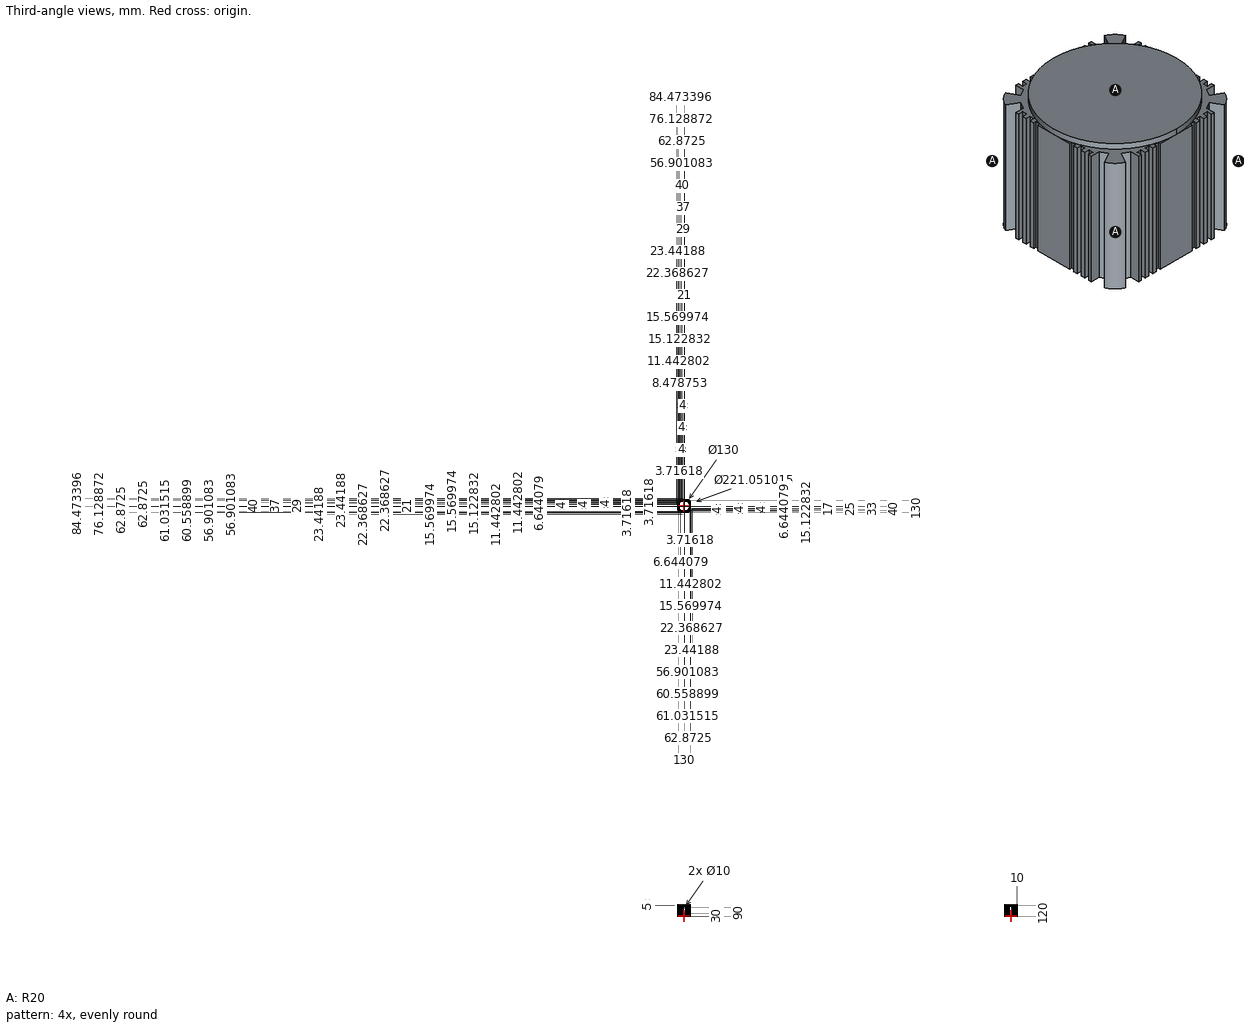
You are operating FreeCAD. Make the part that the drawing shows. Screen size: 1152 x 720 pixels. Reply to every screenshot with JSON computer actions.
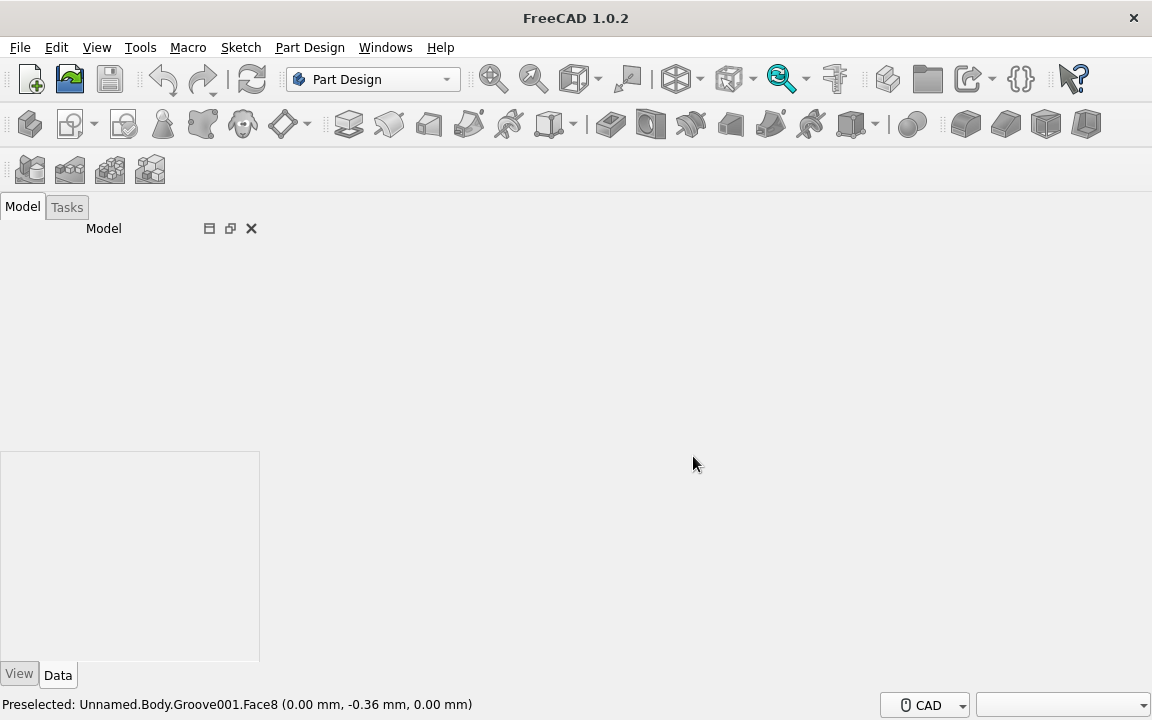
{"action": "key", "text": "ctrl+n"}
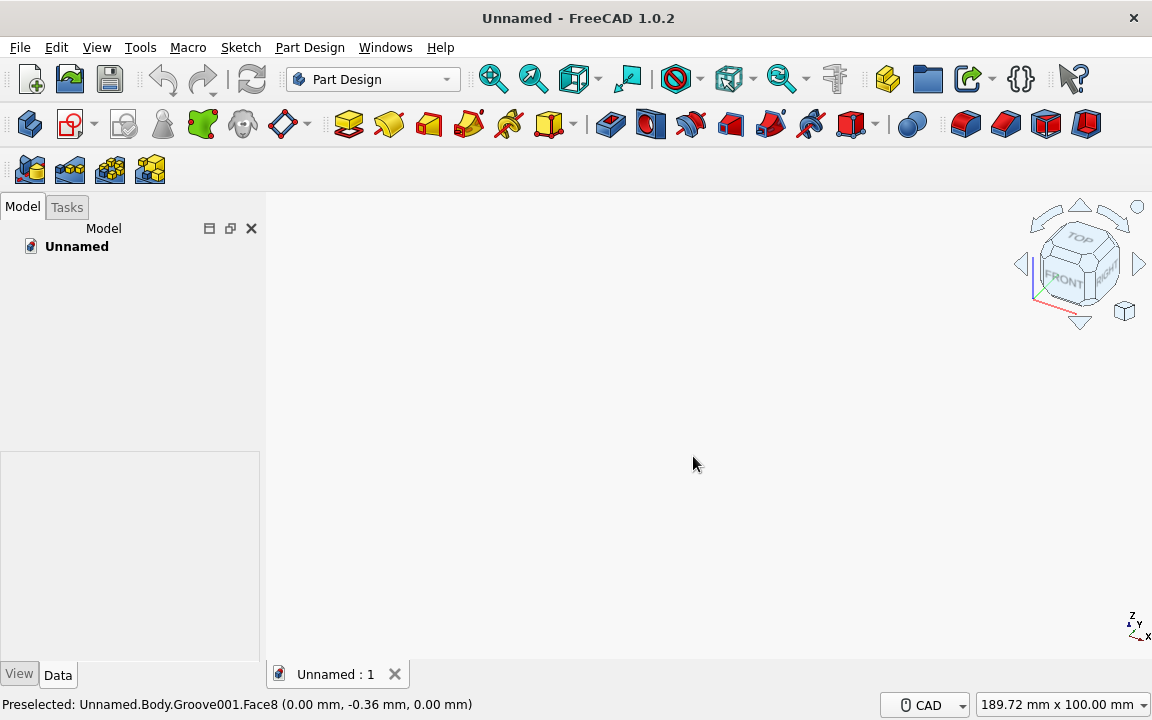
{"action": "left_click", "coordinate": [70, 124]}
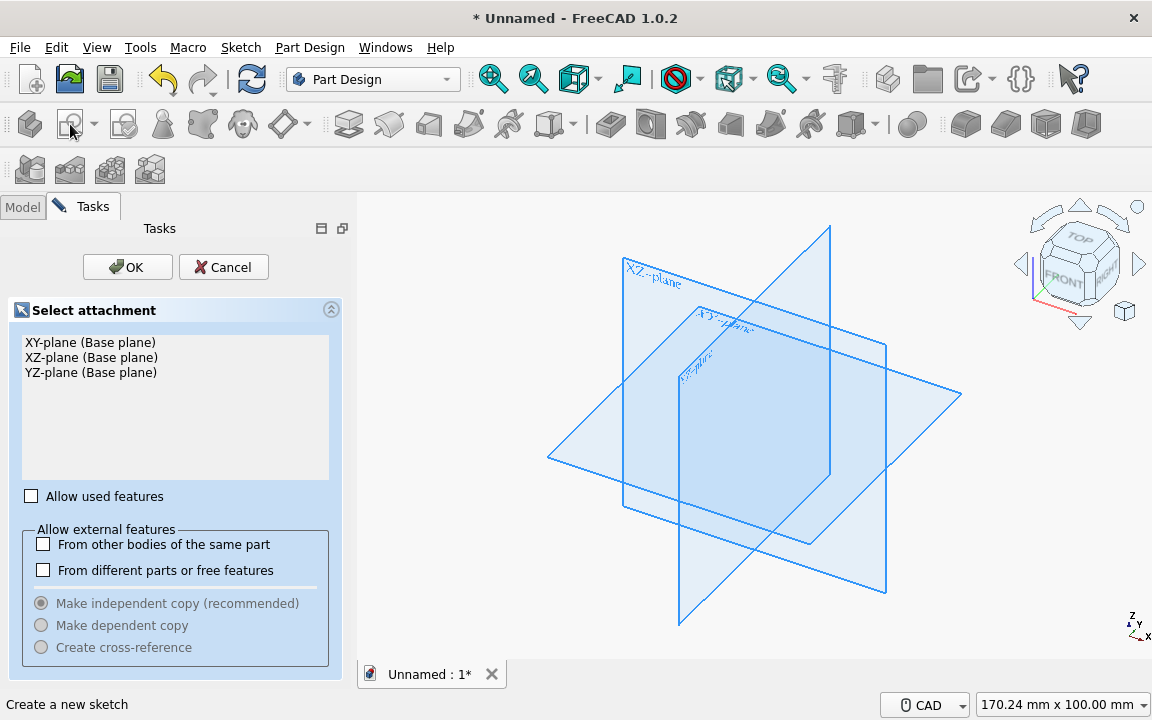
{"action": "left_click", "coordinate": [82, 342]}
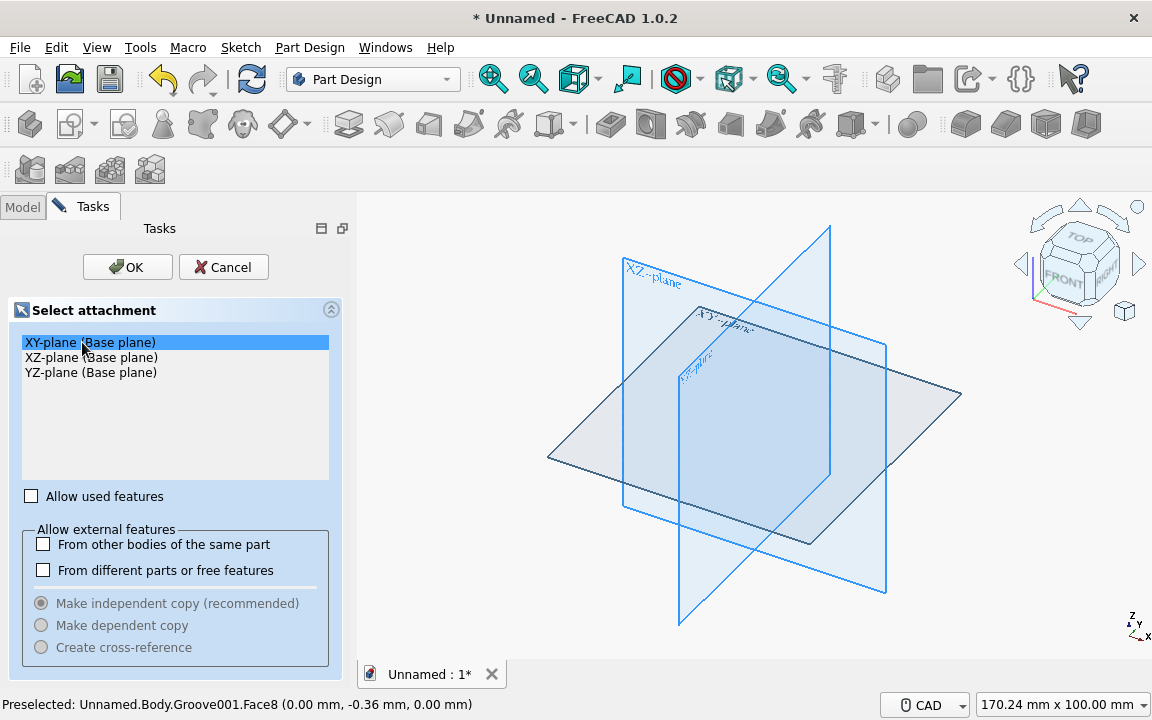
{"action": "left_click", "coordinate": [128, 267]}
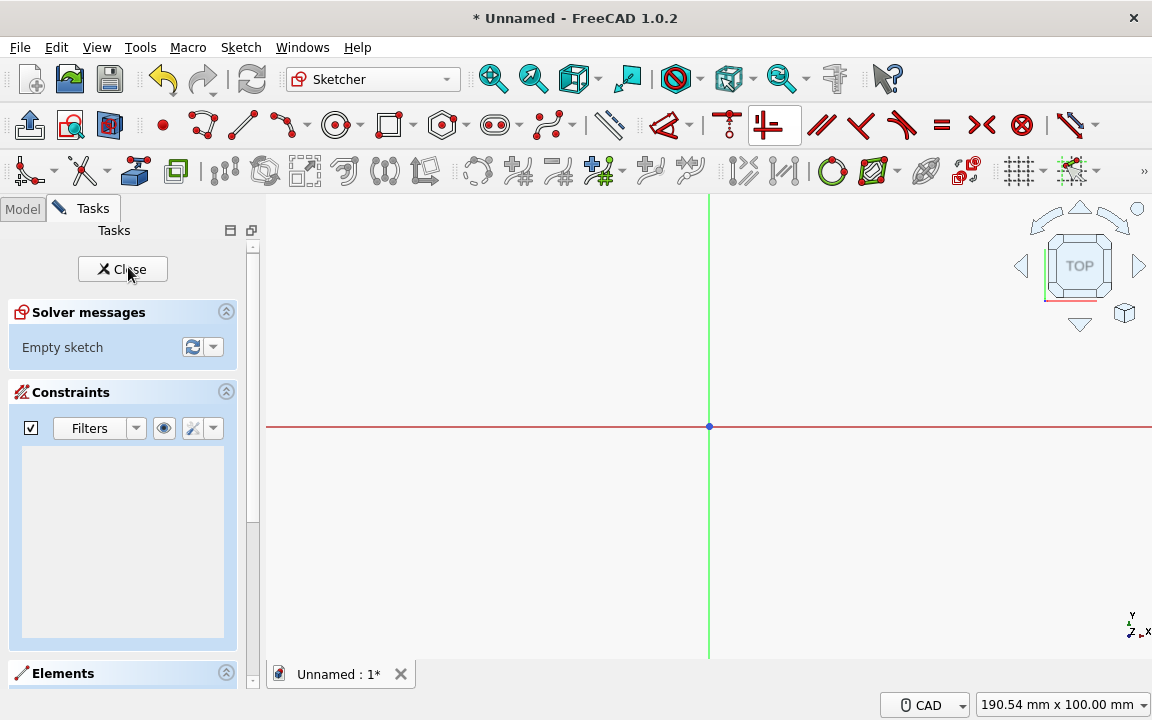
{"action": "scroll", "coordinate": [585, 426], "scroll_direction": "down", "scroll_amount": 4}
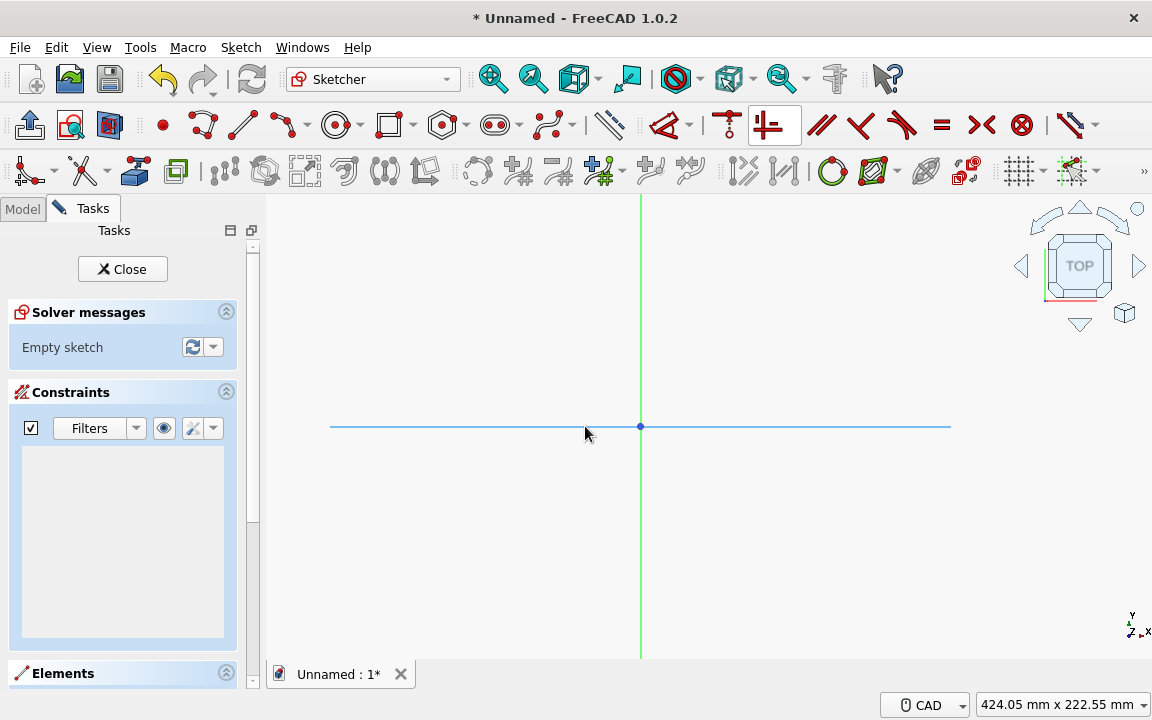
{"action": "key", "text": "g v"}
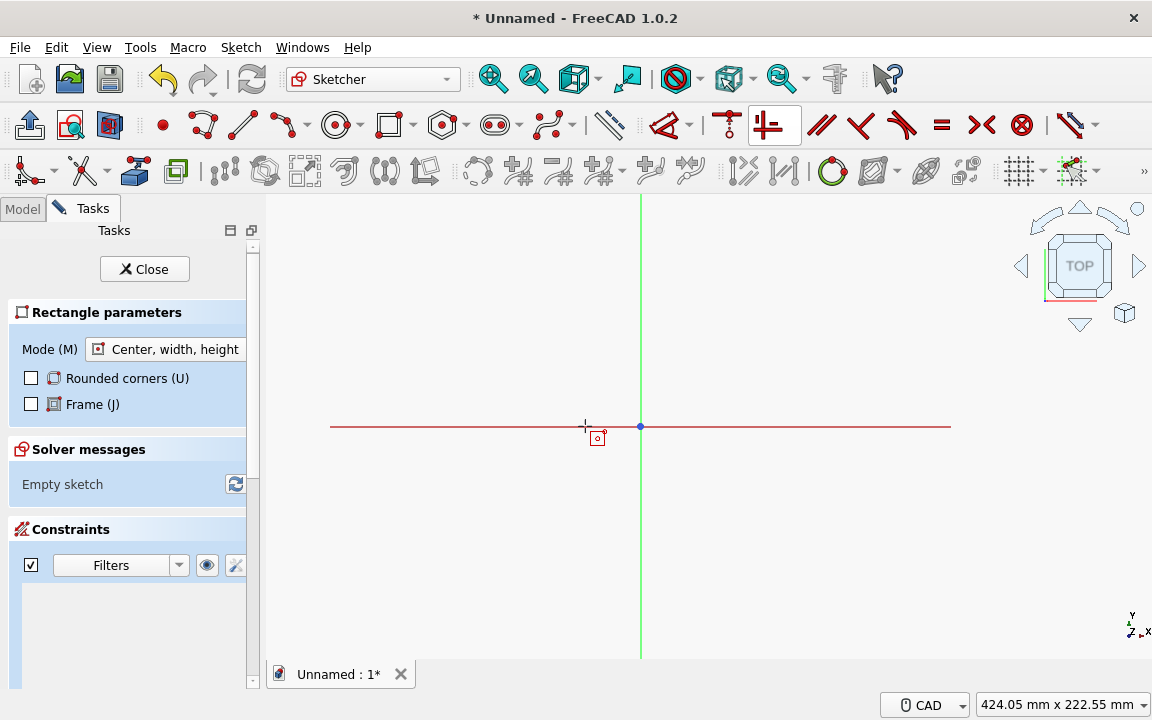
{"action": "left_click", "coordinate": [641, 426]}
{"action": "mouse_move", "coordinate": [777, 291]}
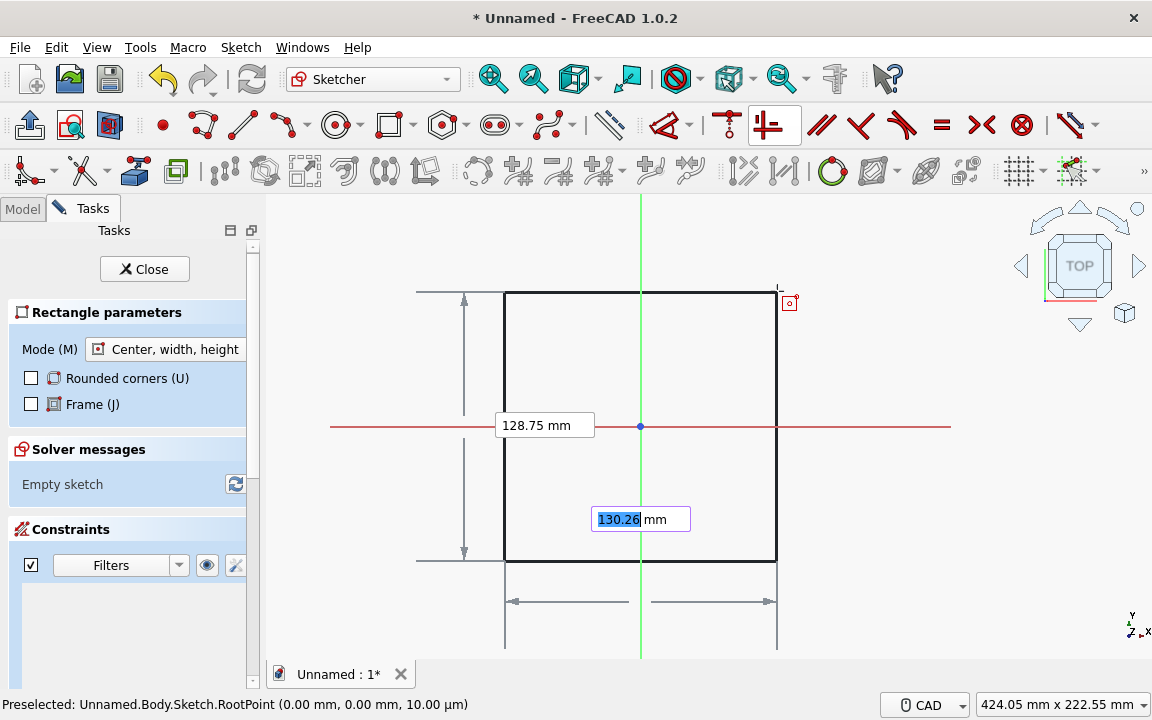
{"action": "type", "text": "130"}
{"action": "key", "text": "Tab"}
{"action": "type", "text": "130"}
{"action": "key", "text": "Return"}
{"action": "key", "text": "Escape"}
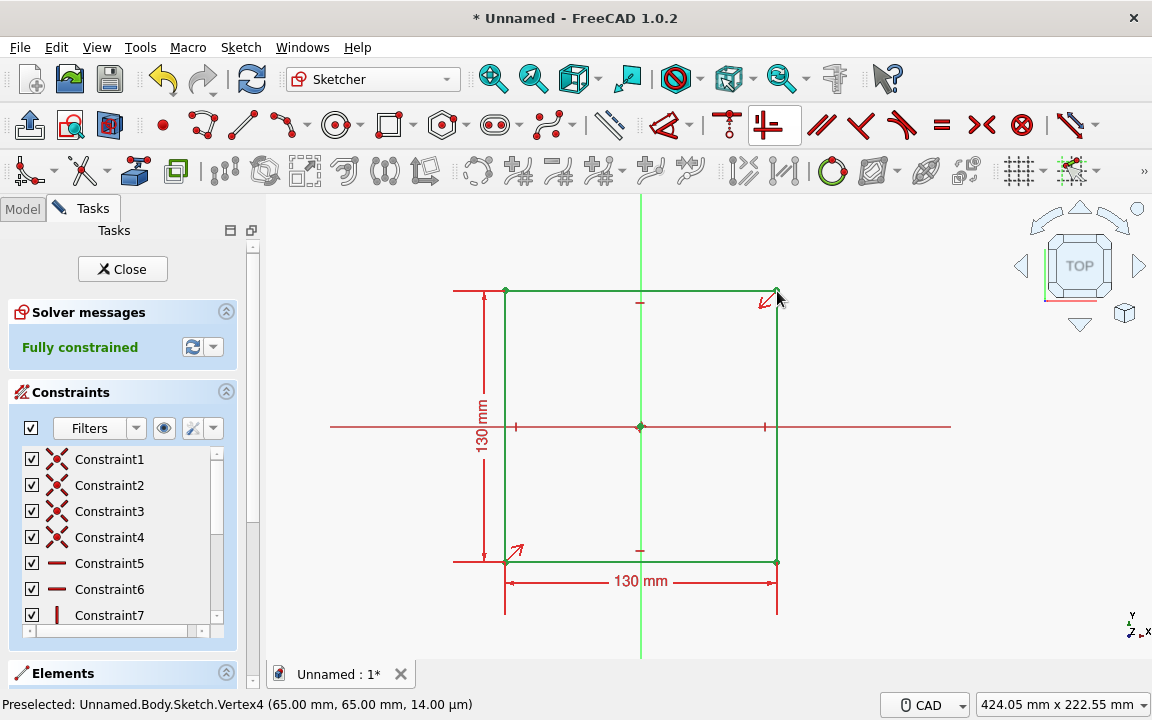
{"action": "left_click", "coordinate": [123, 269]}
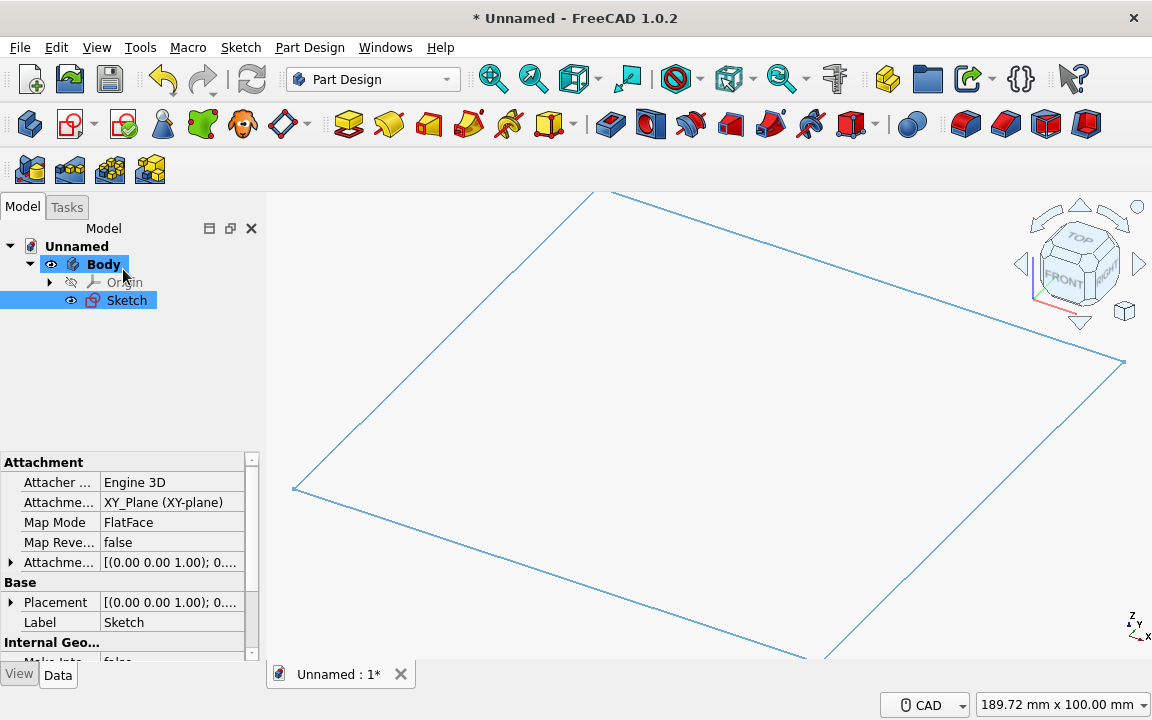
{"action": "left_click", "coordinate": [350, 124]}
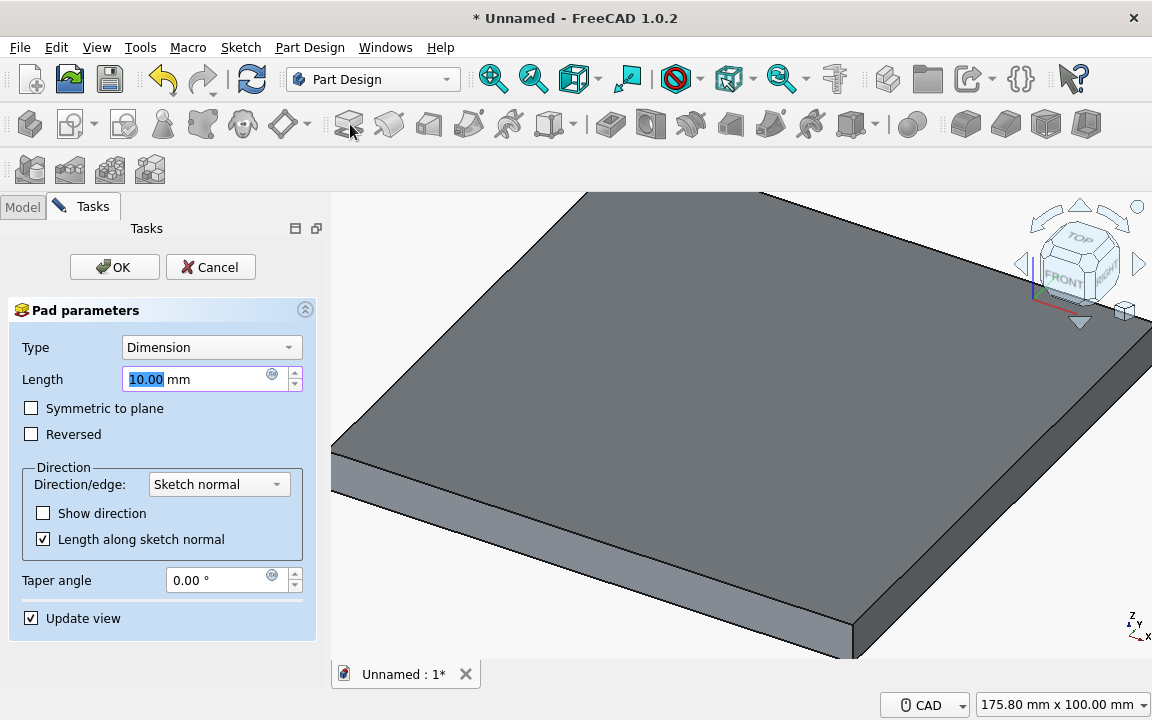
{"action": "type", "text": "120"}
{"action": "key", "text": "Tab"}